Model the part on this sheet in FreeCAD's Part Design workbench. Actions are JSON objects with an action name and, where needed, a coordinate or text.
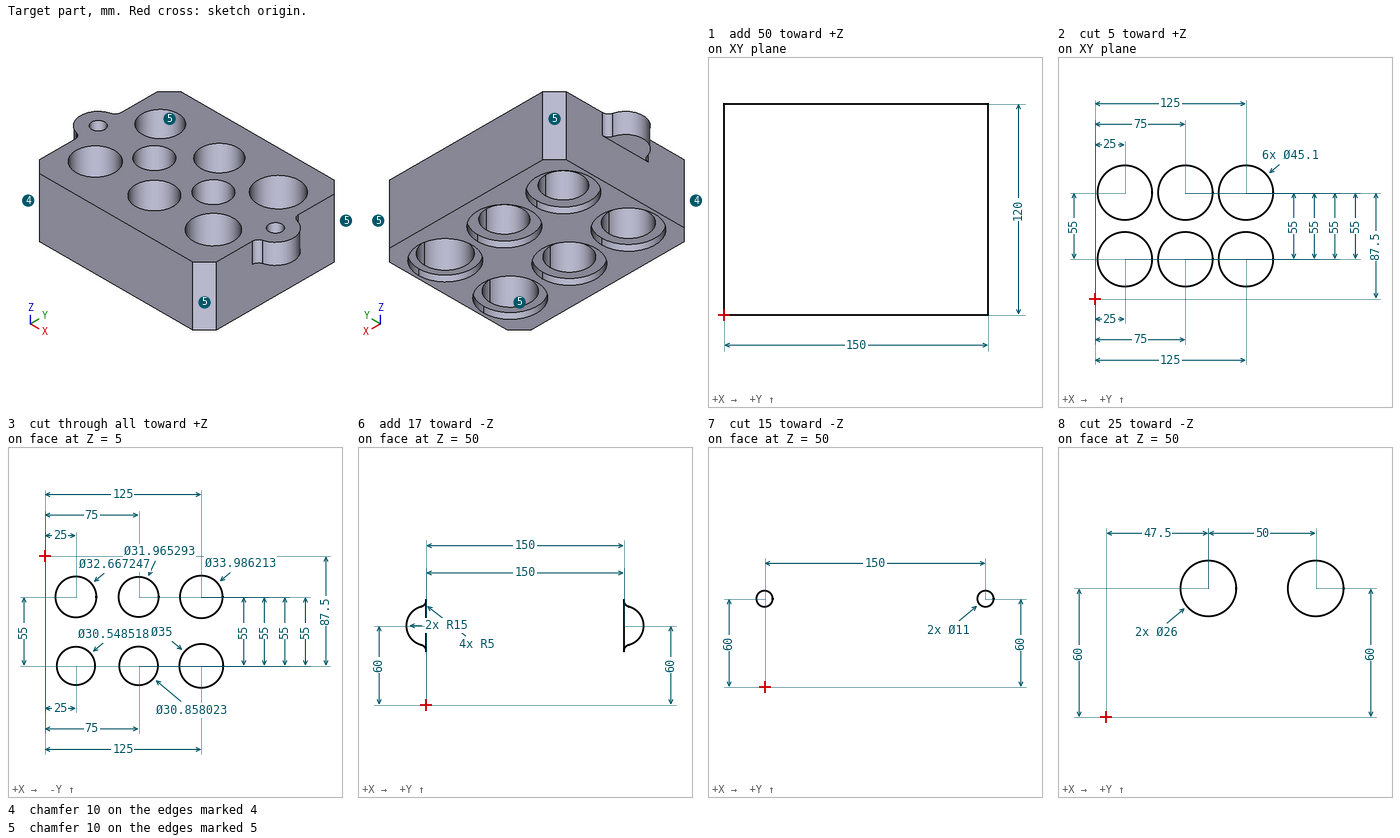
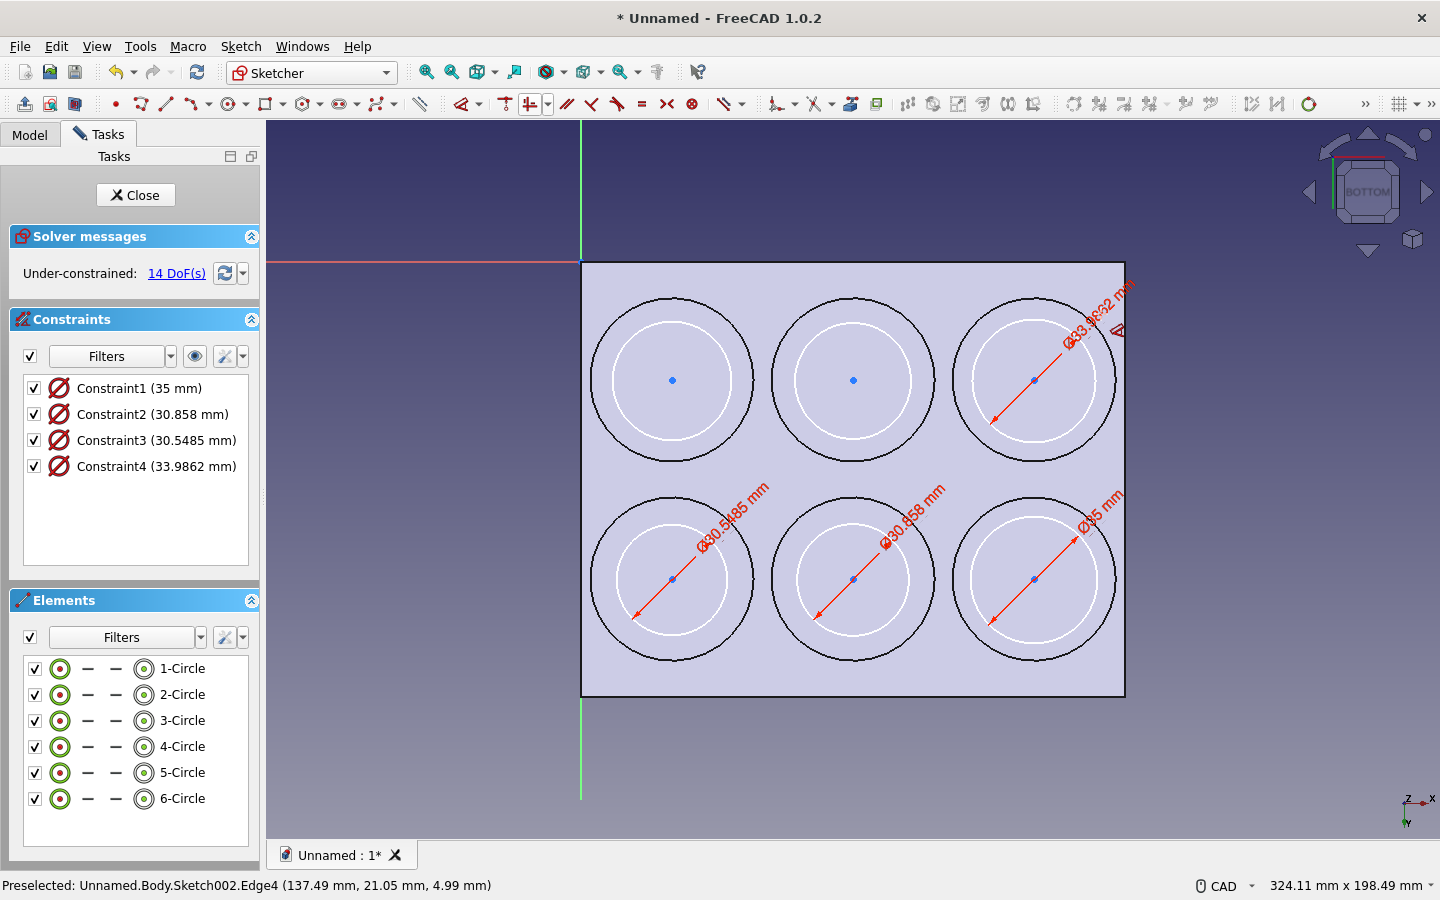
{"action": "left_click", "coordinate": [894, 340]}
{"action": "left_click", "coordinate": [917, 317]}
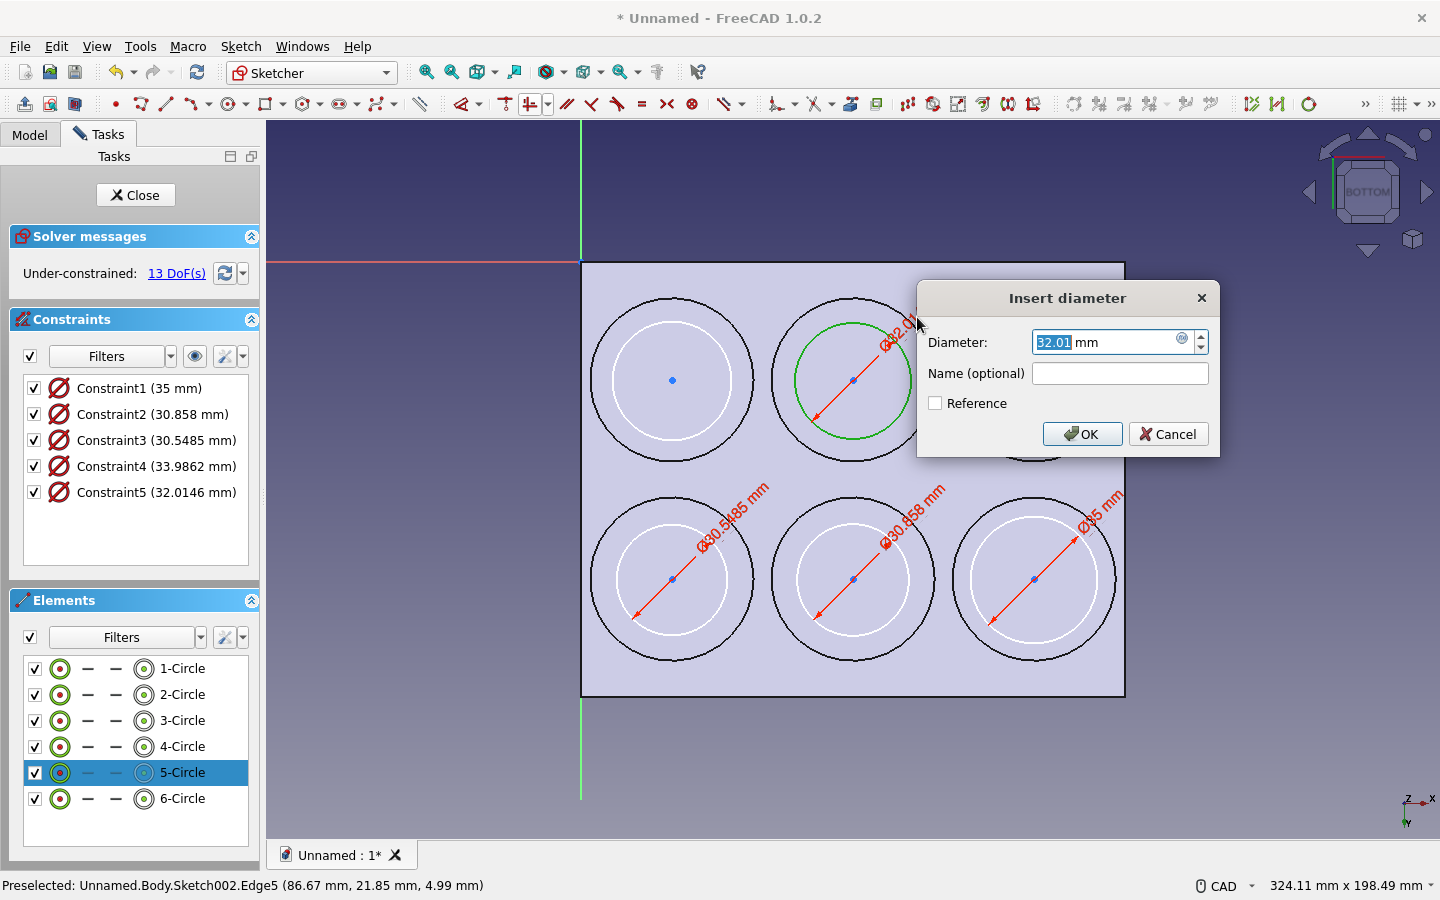
{"action": "type", "text": "31.965293"}
{"action": "key", "text": "Return"}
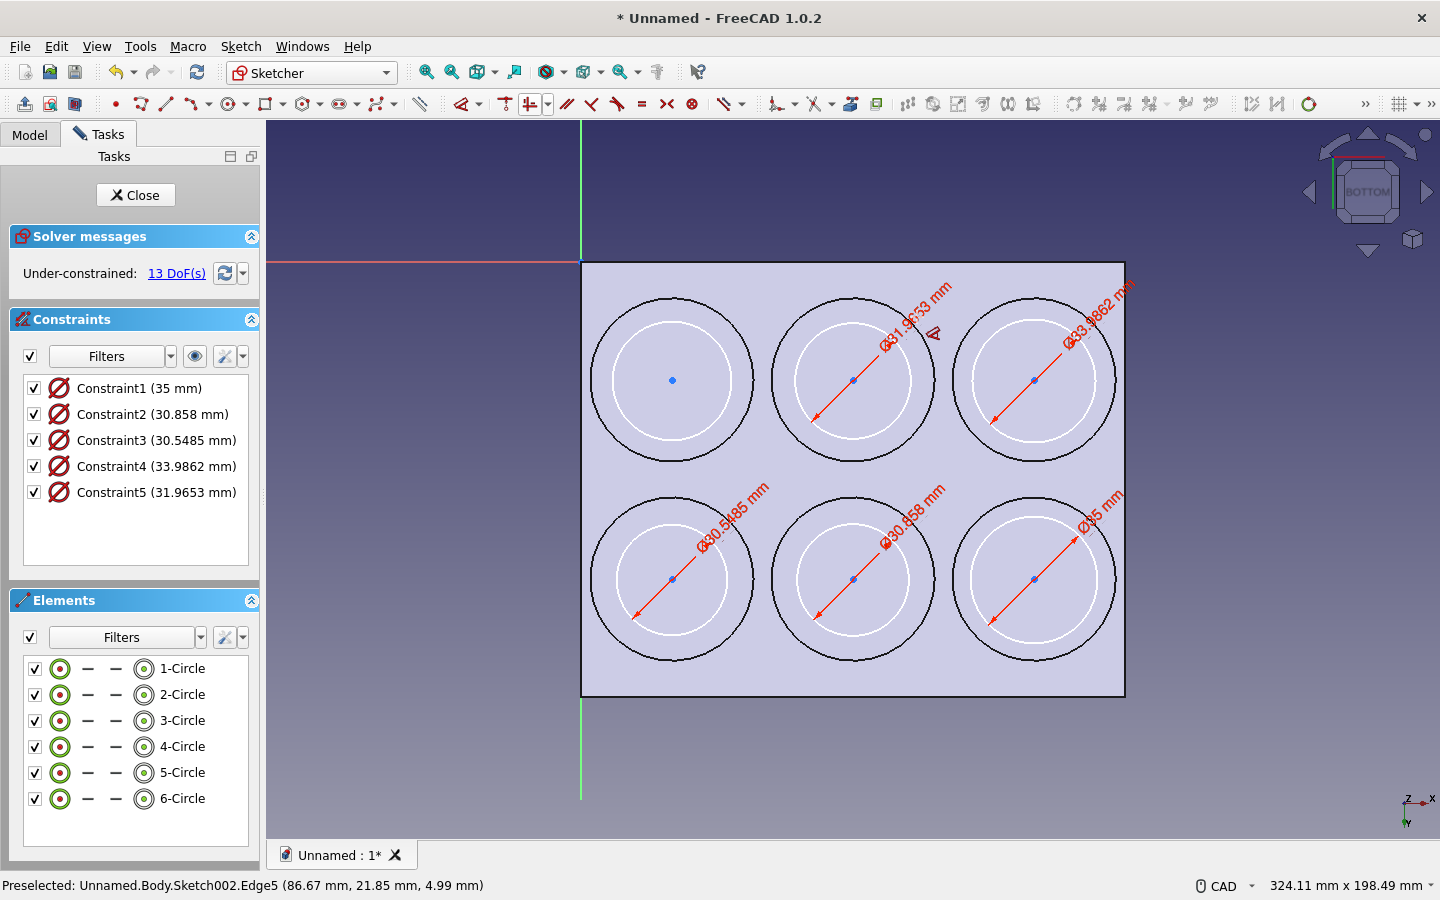
{"action": "left_click", "coordinate": [714, 339]}
{"action": "left_click", "coordinate": [737, 316]}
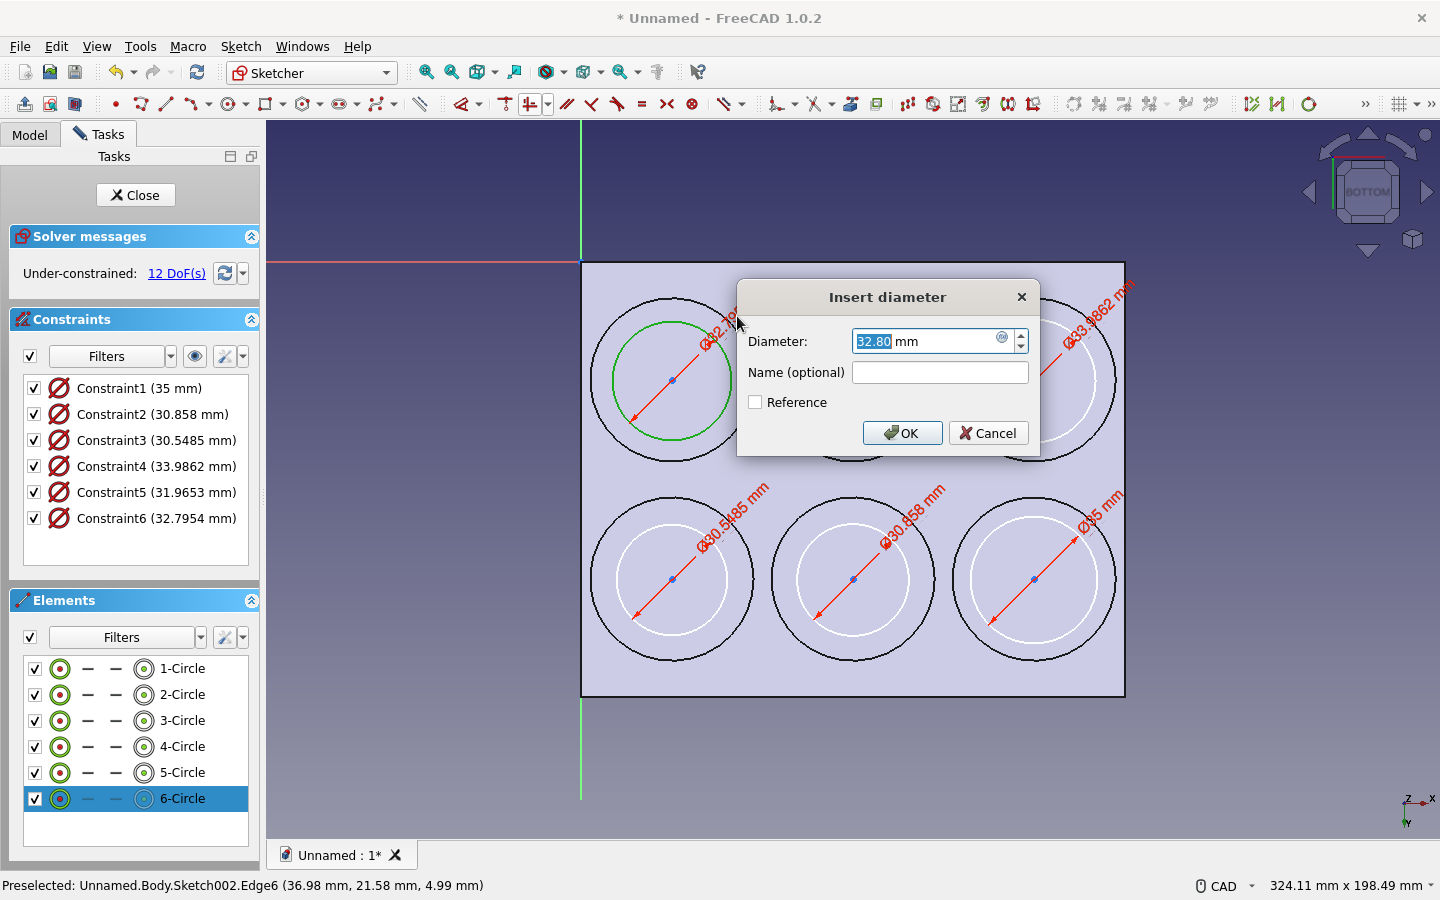
{"action": "type", "text": "32.667247"}
{"action": "key", "text": "Return"}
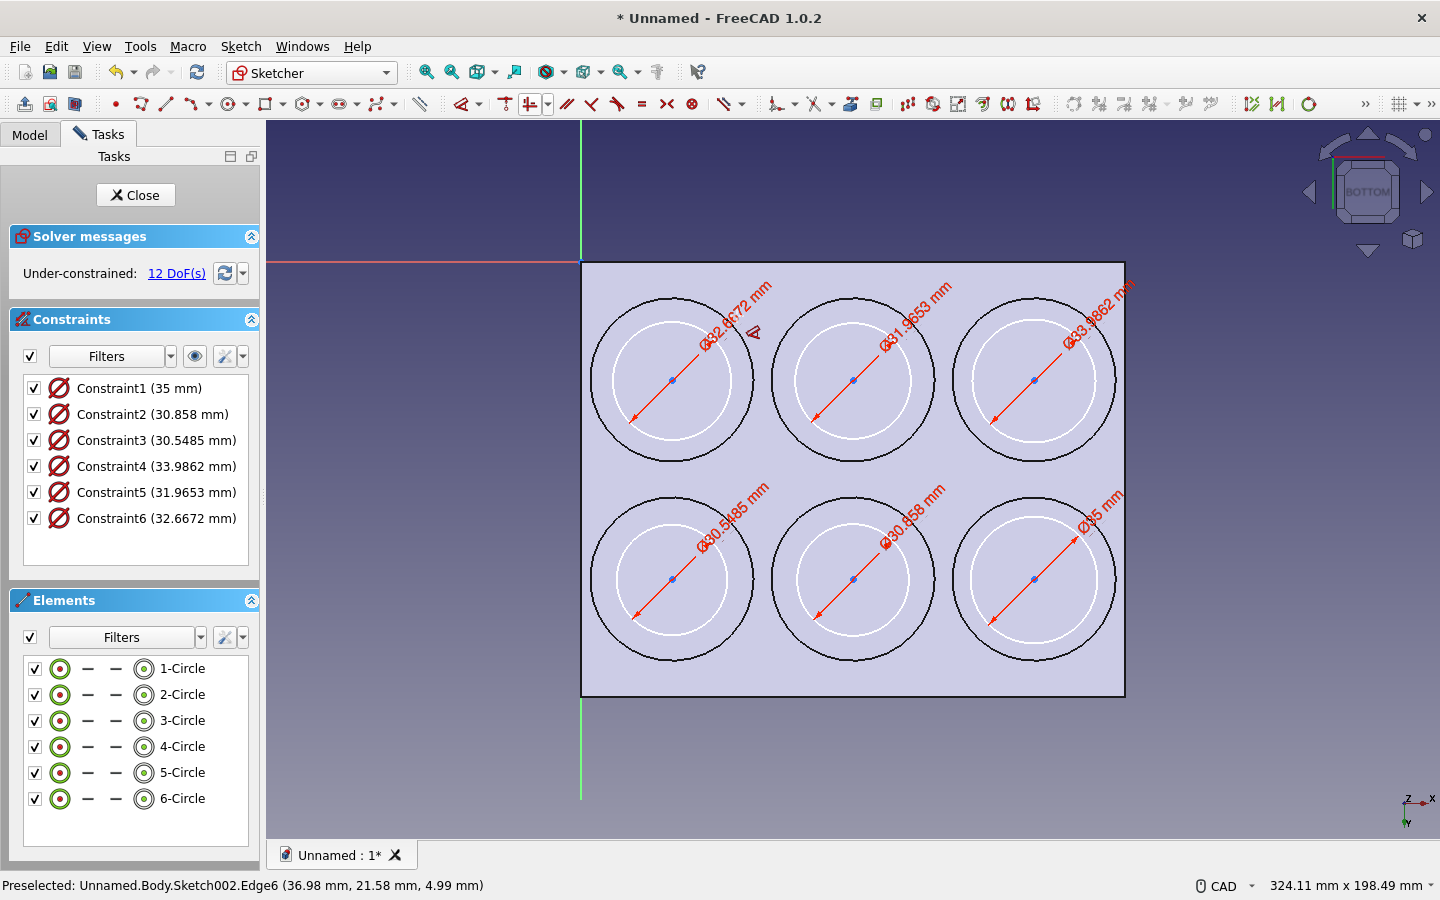
{"action": "left_click", "coordinate": [853, 580]}
{"action": "left_click", "coordinate": [717, 228]}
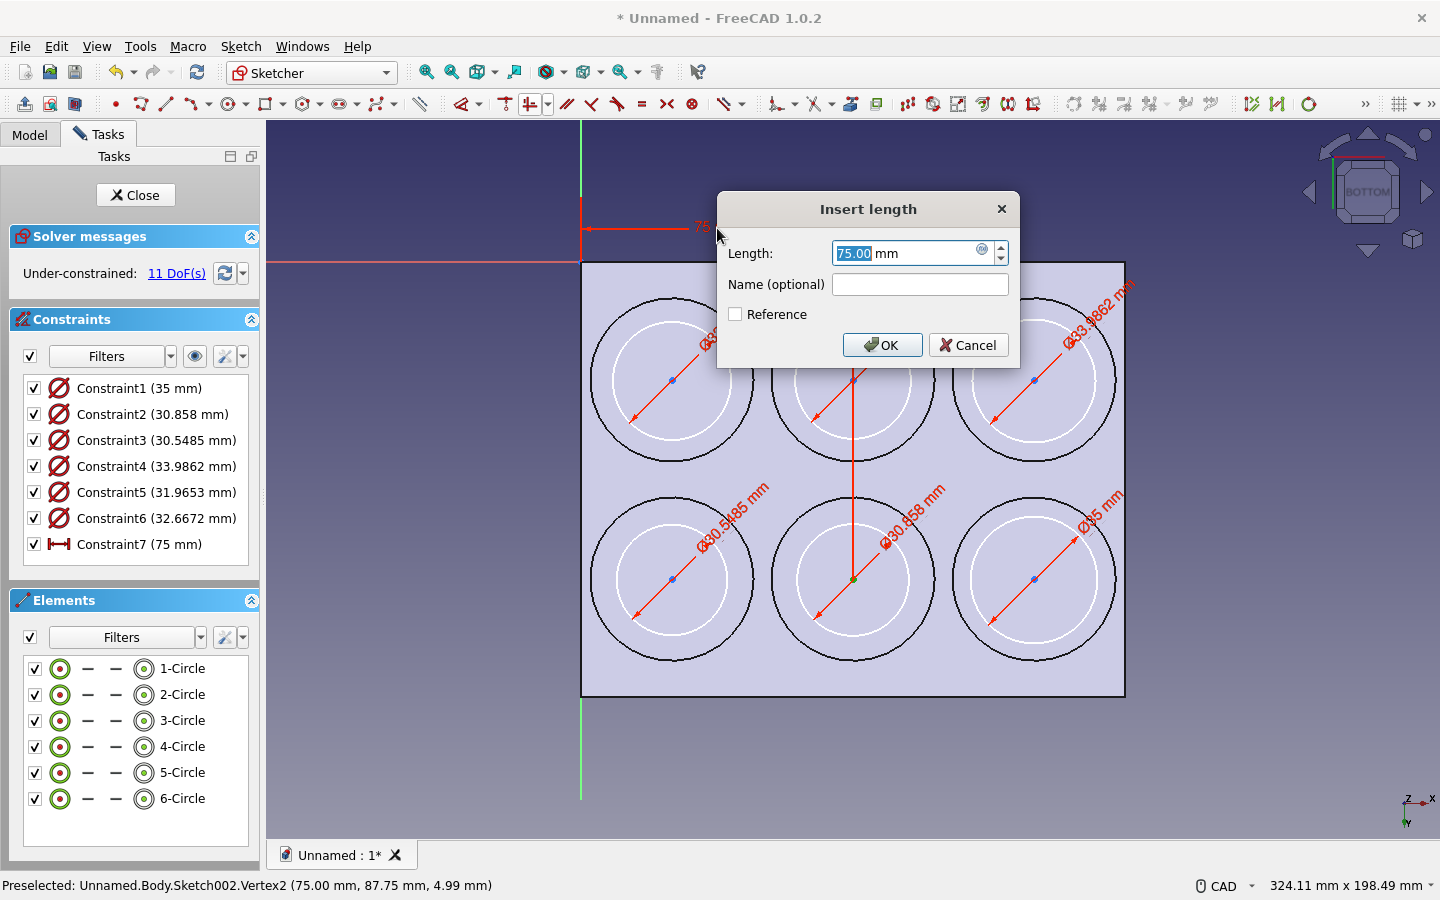
{"action": "type", "text": "75"}
{"action": "key", "text": "Return"}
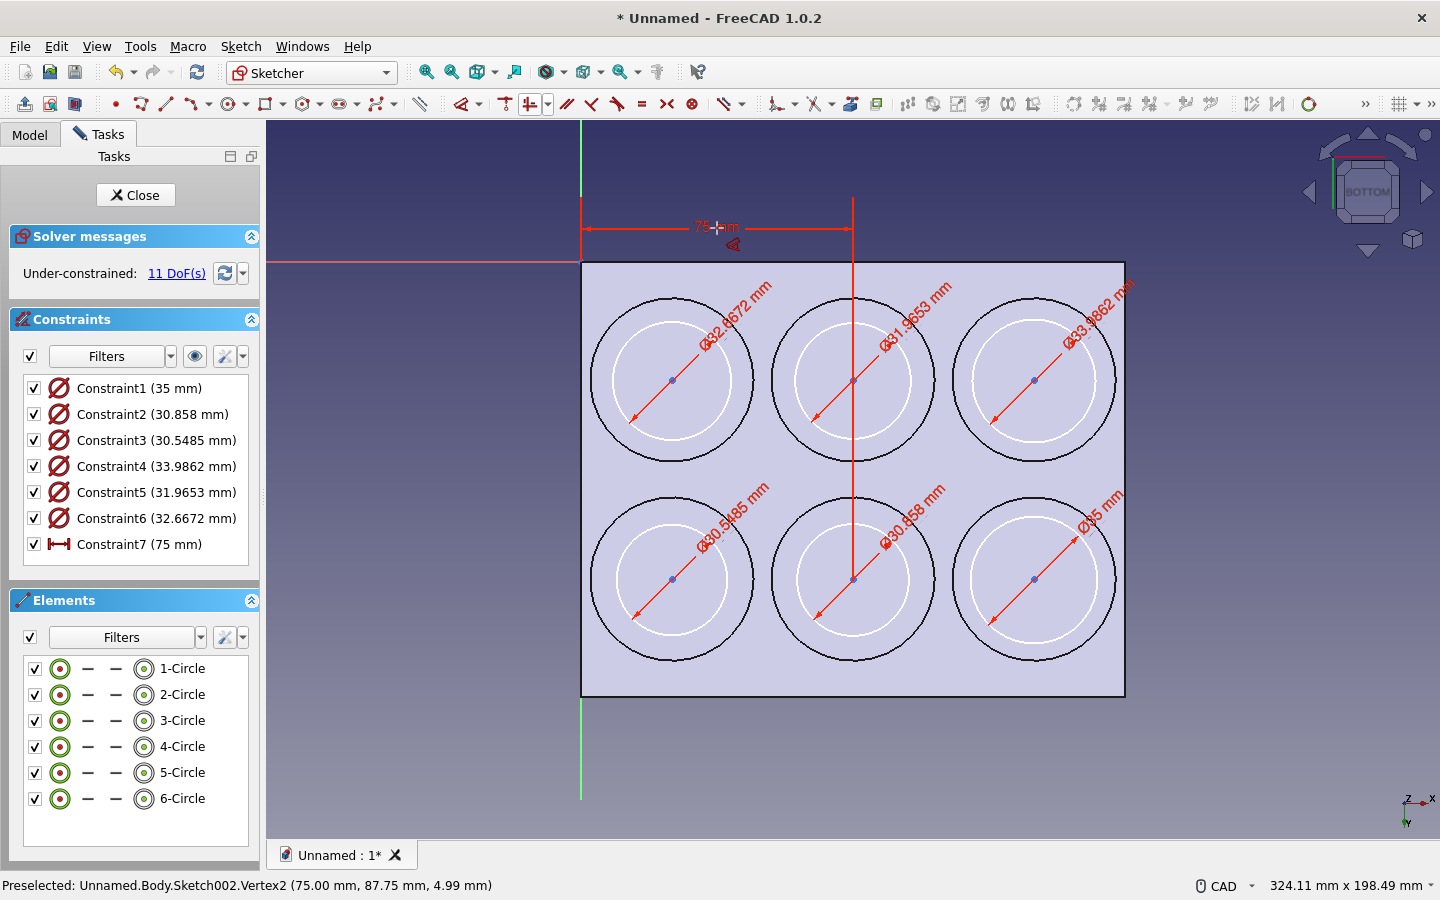
{"action": "left_click", "coordinate": [672, 580]}
{"action": "left_click", "coordinate": [627, 228]}